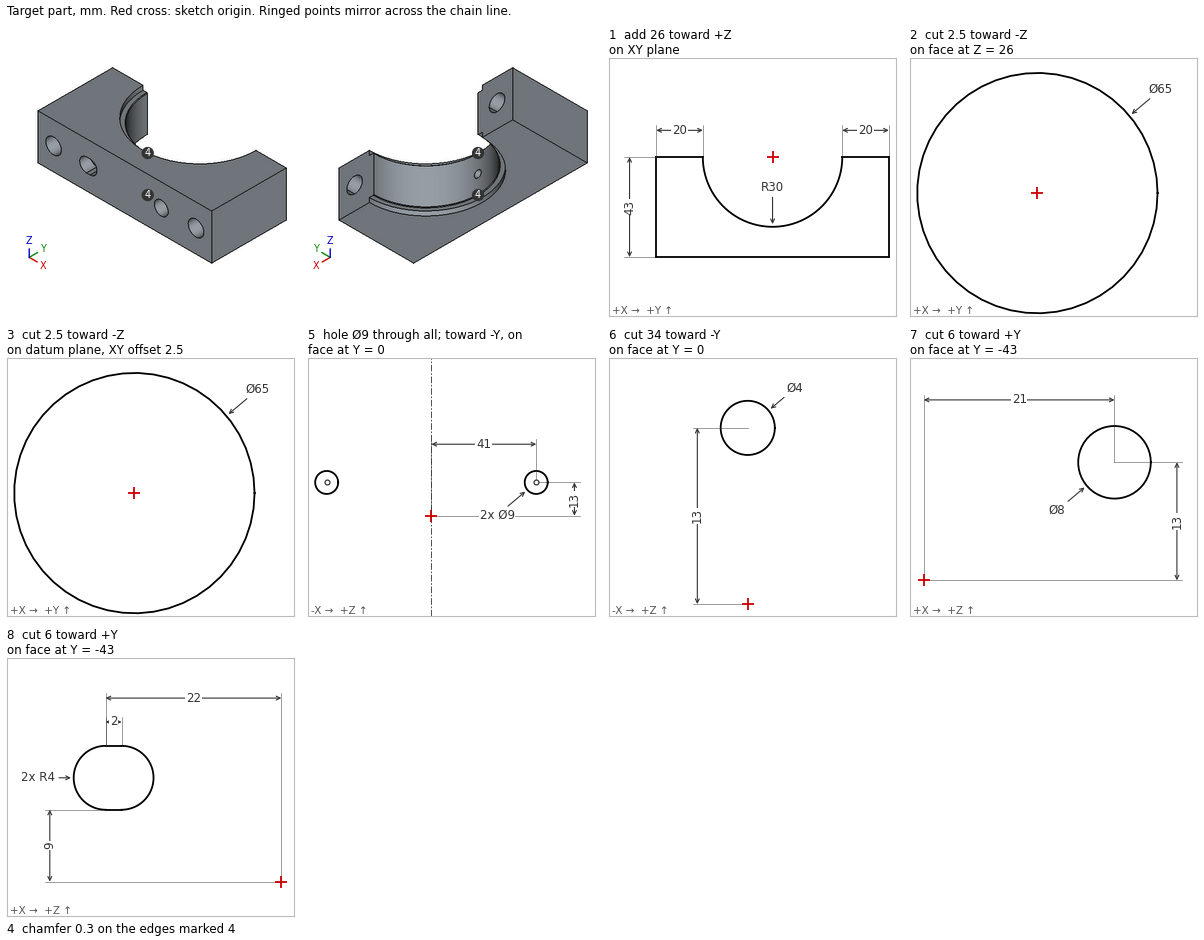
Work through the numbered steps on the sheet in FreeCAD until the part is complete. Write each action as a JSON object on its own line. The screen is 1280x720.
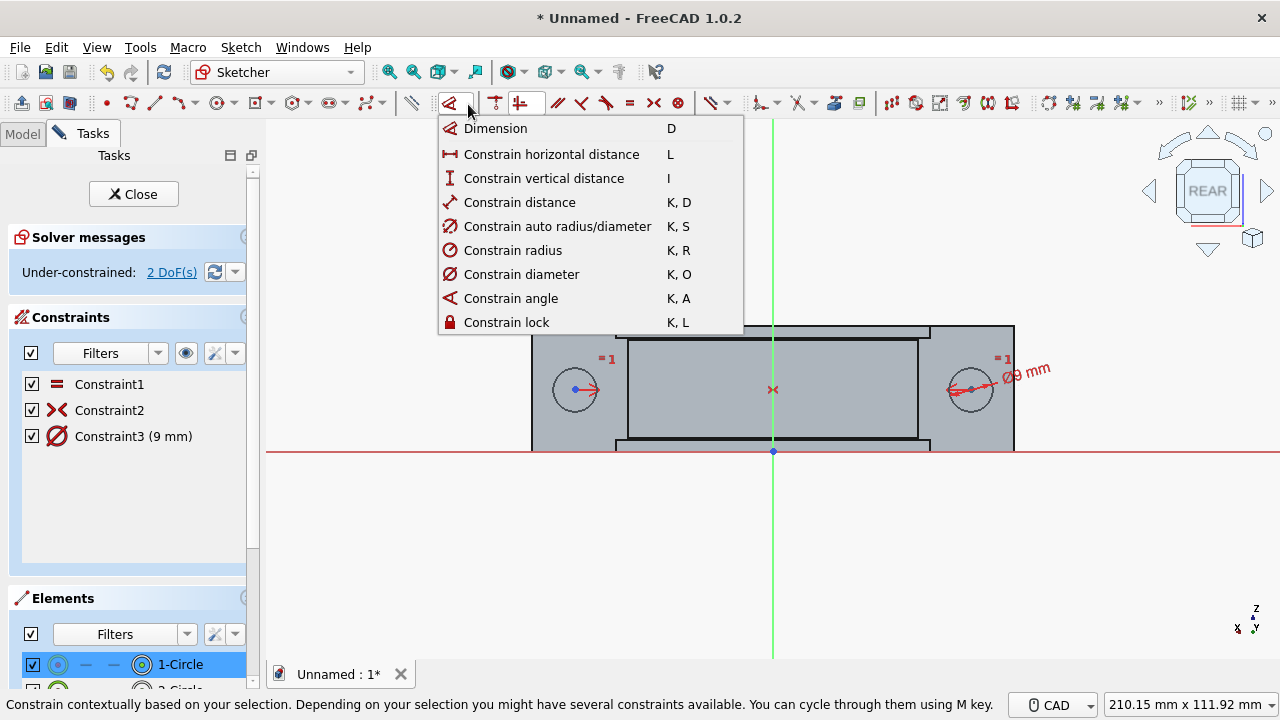
{"action": "left_click", "coordinate": [591, 154]}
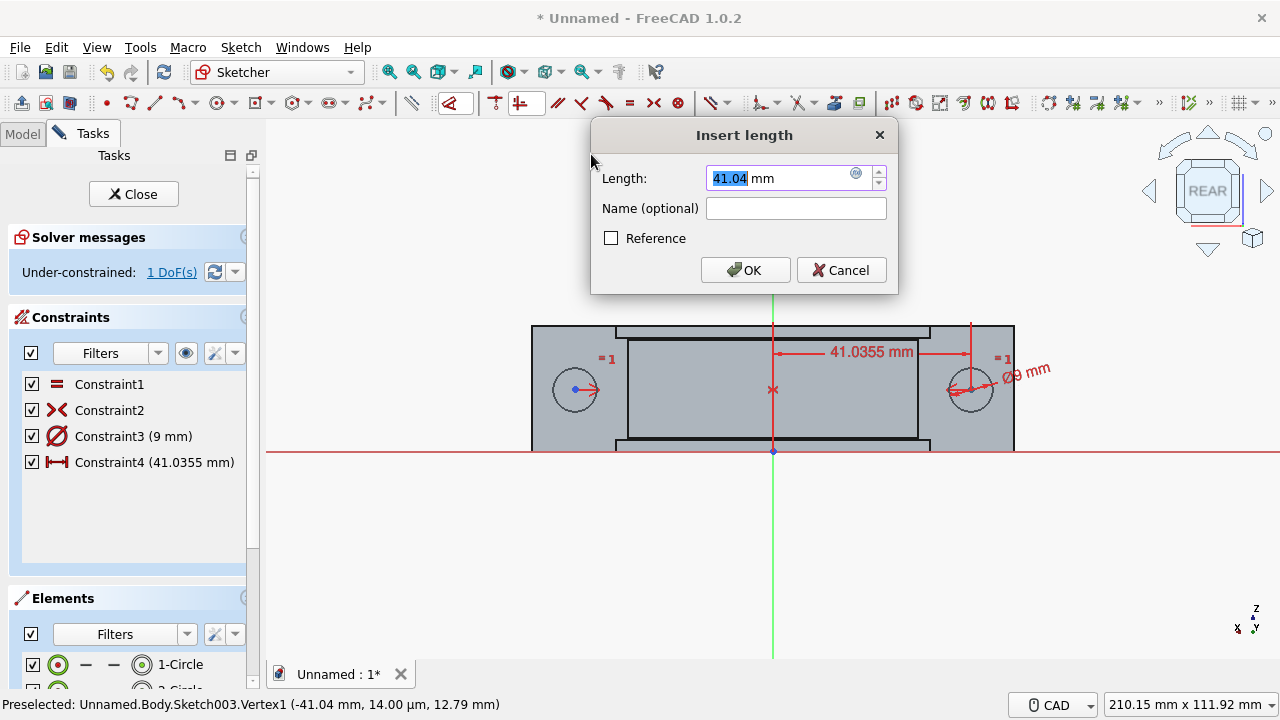
{"action": "type", "text": "41"}
{"action": "key", "text": "Return"}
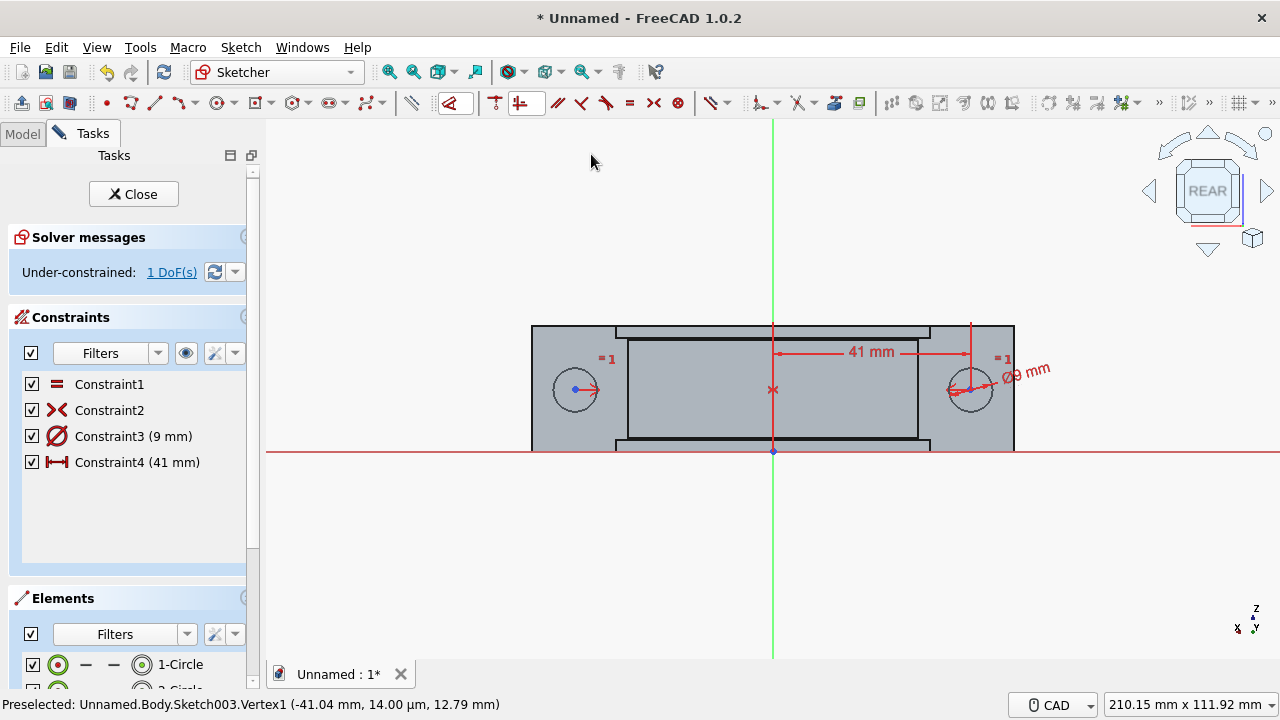
{"action": "left_click", "coordinate": [971, 390]}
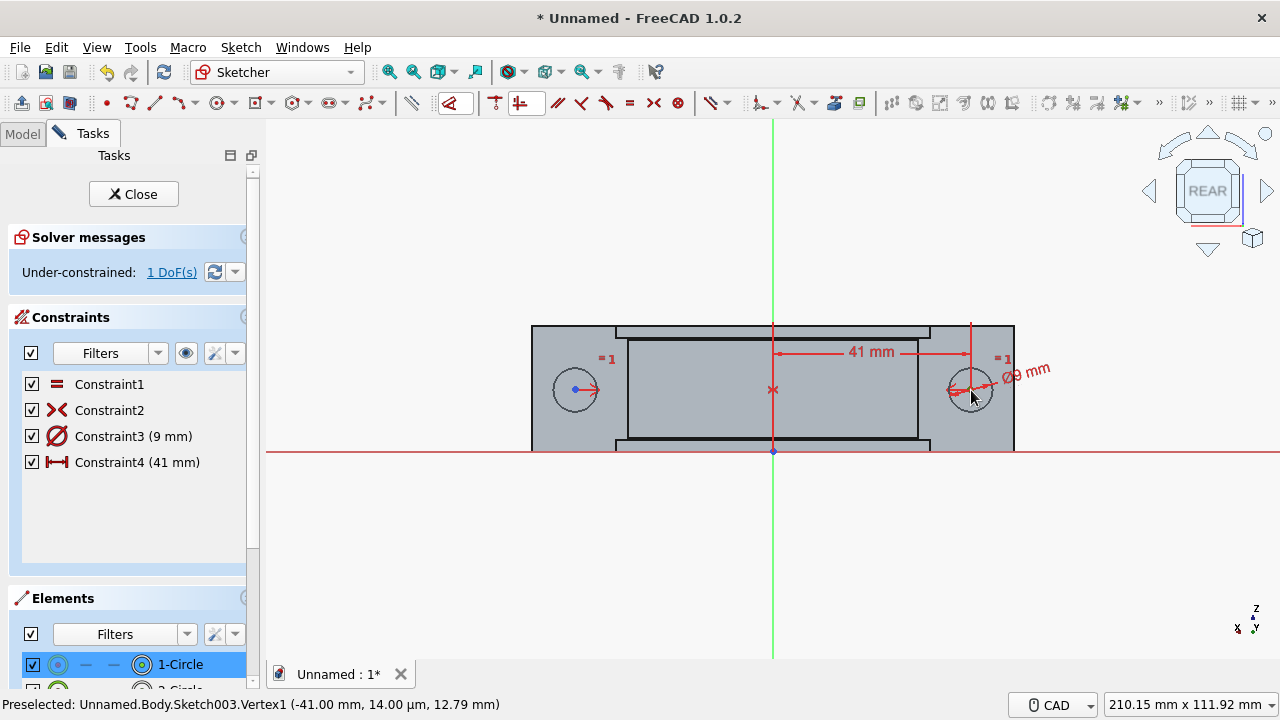
{"action": "left_click", "coordinate": [468, 104]}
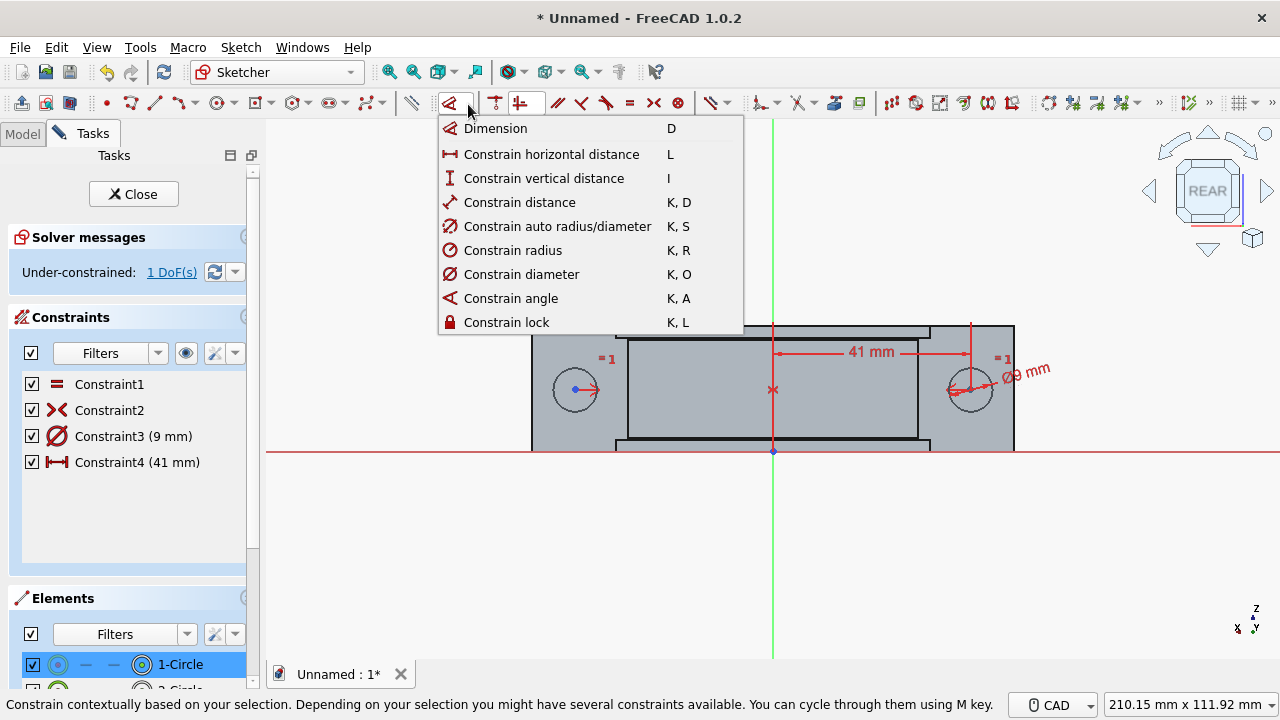
{"action": "left_click", "coordinate": [591, 178]}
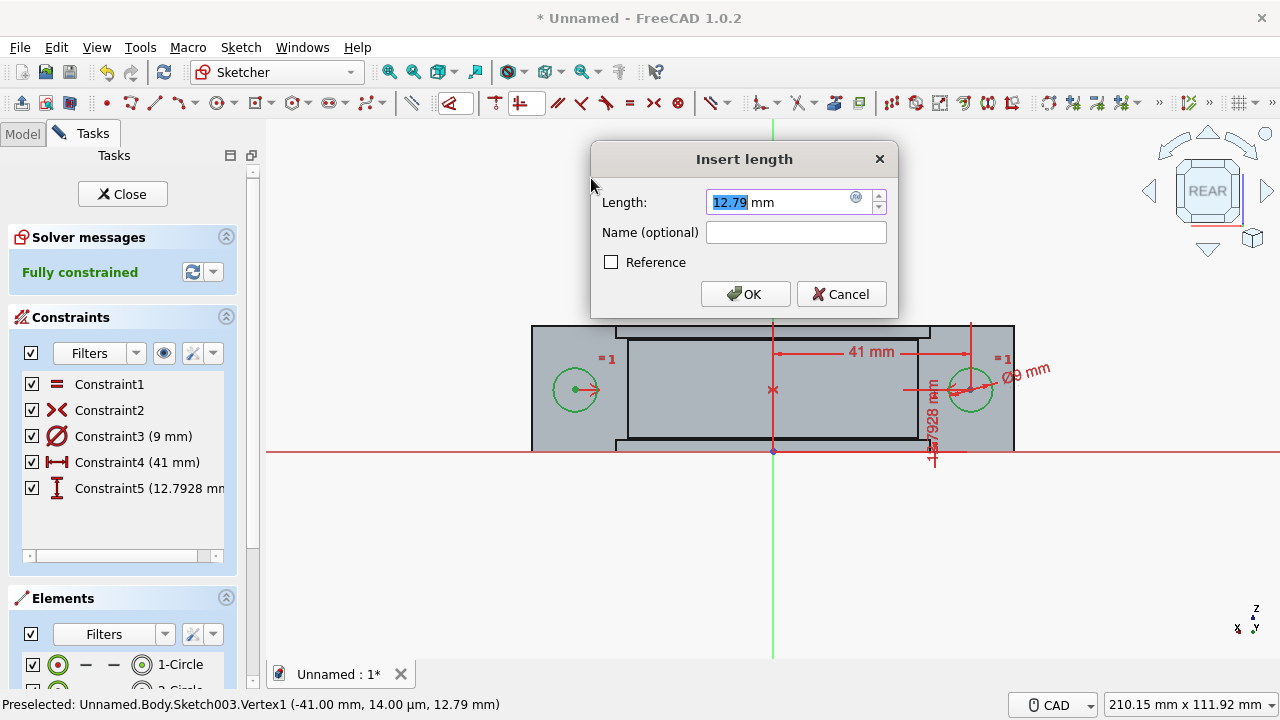
{"action": "type", "text": "13"}
{"action": "key", "text": "Return"}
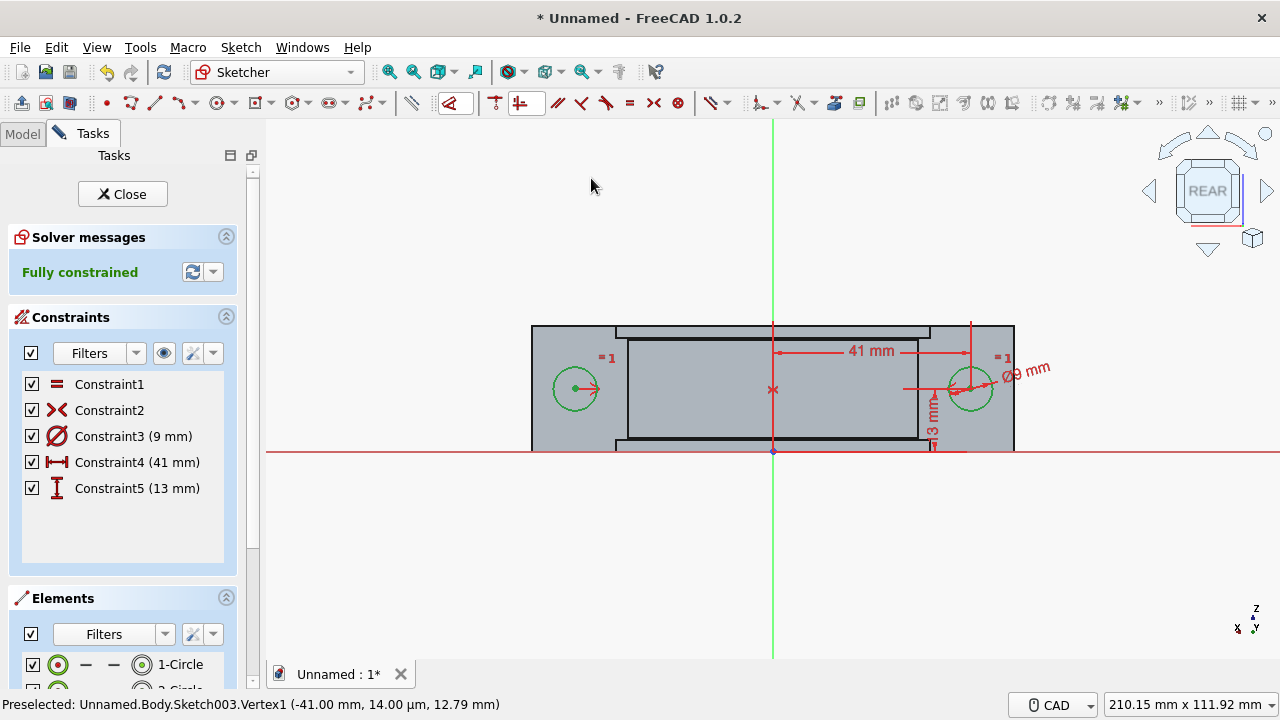
{"action": "left_click", "coordinate": [123, 194]}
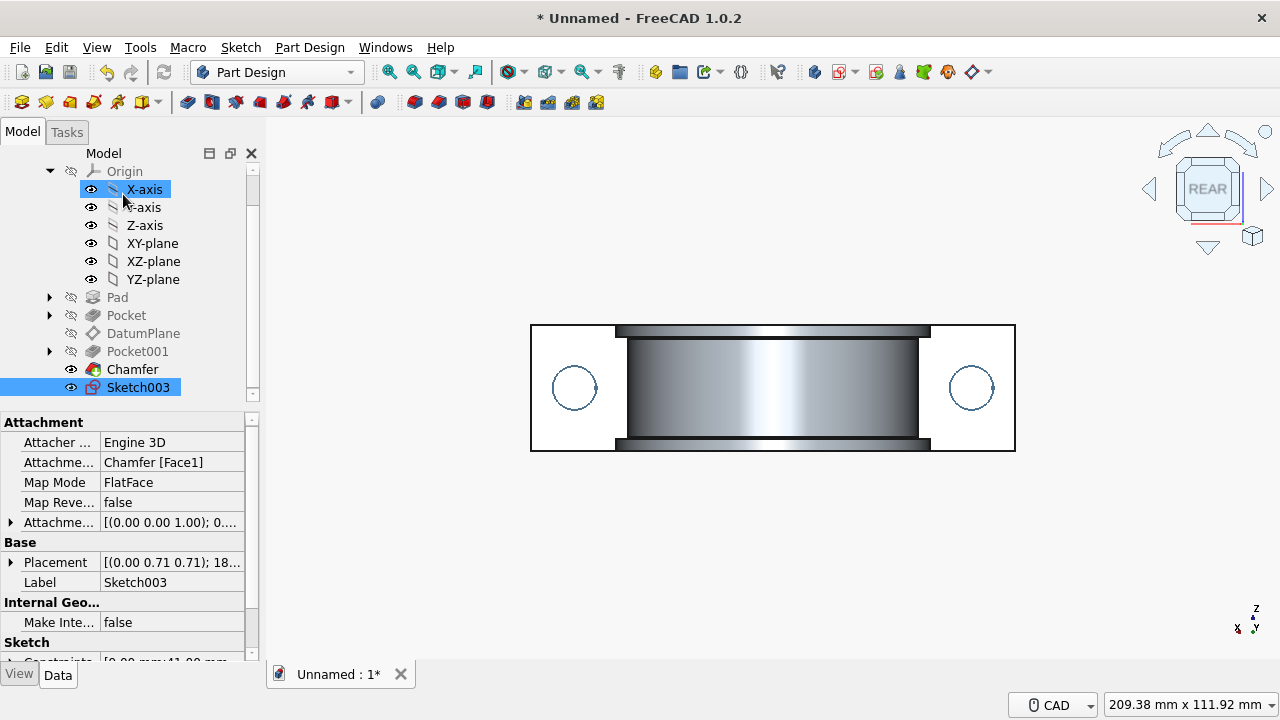
{"action": "left_click", "coordinate": [212, 102]}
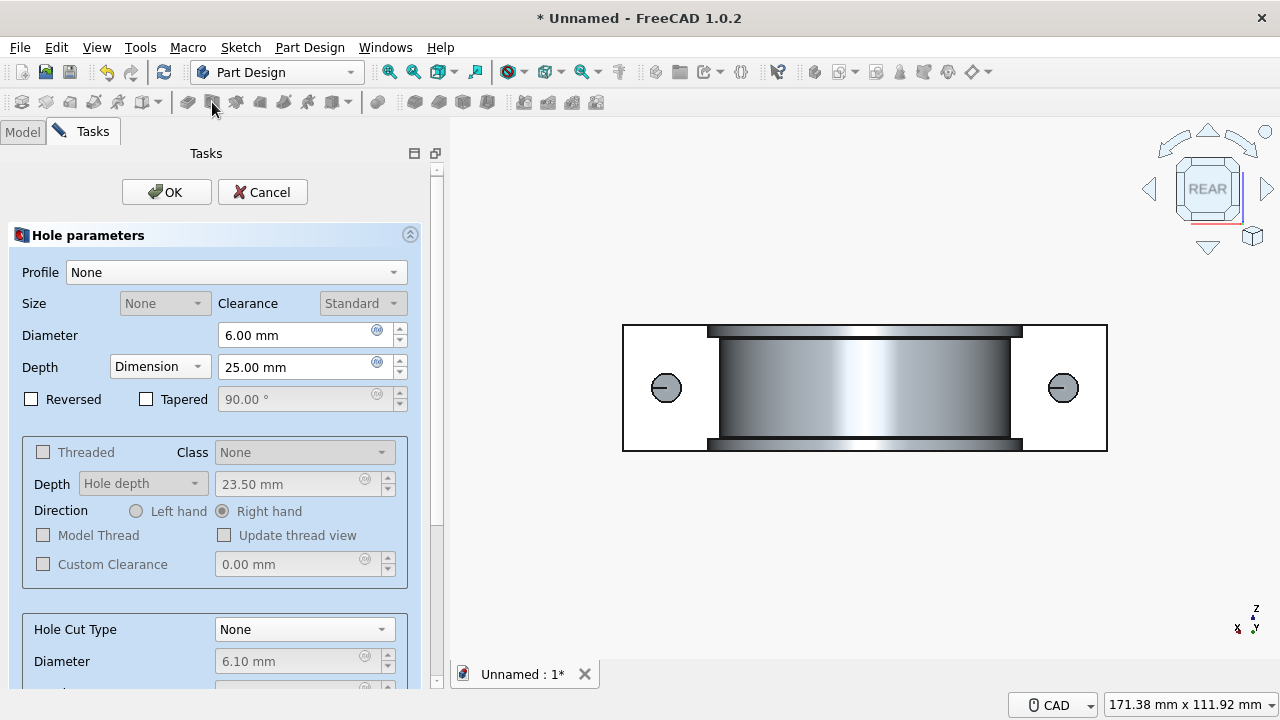
{"action": "triple_click", "coordinate": [305, 335]}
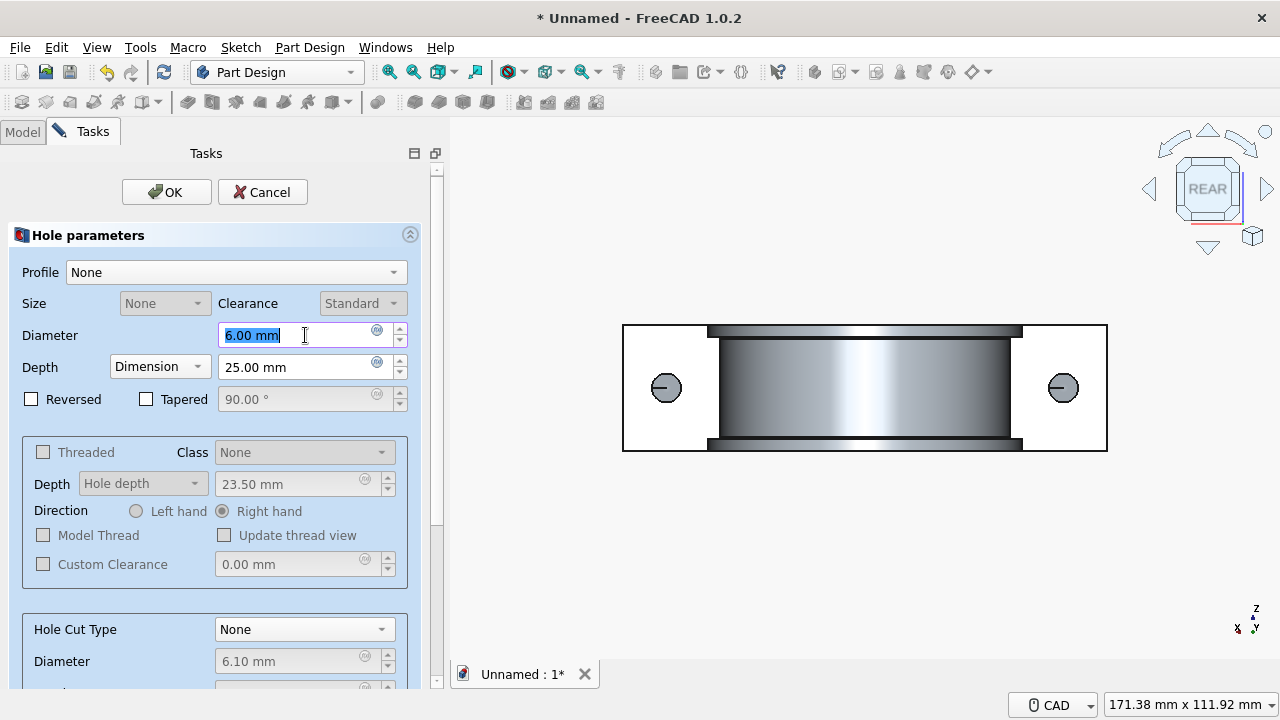
{"action": "type", "text": "9"}
{"action": "key", "text": "Tab"}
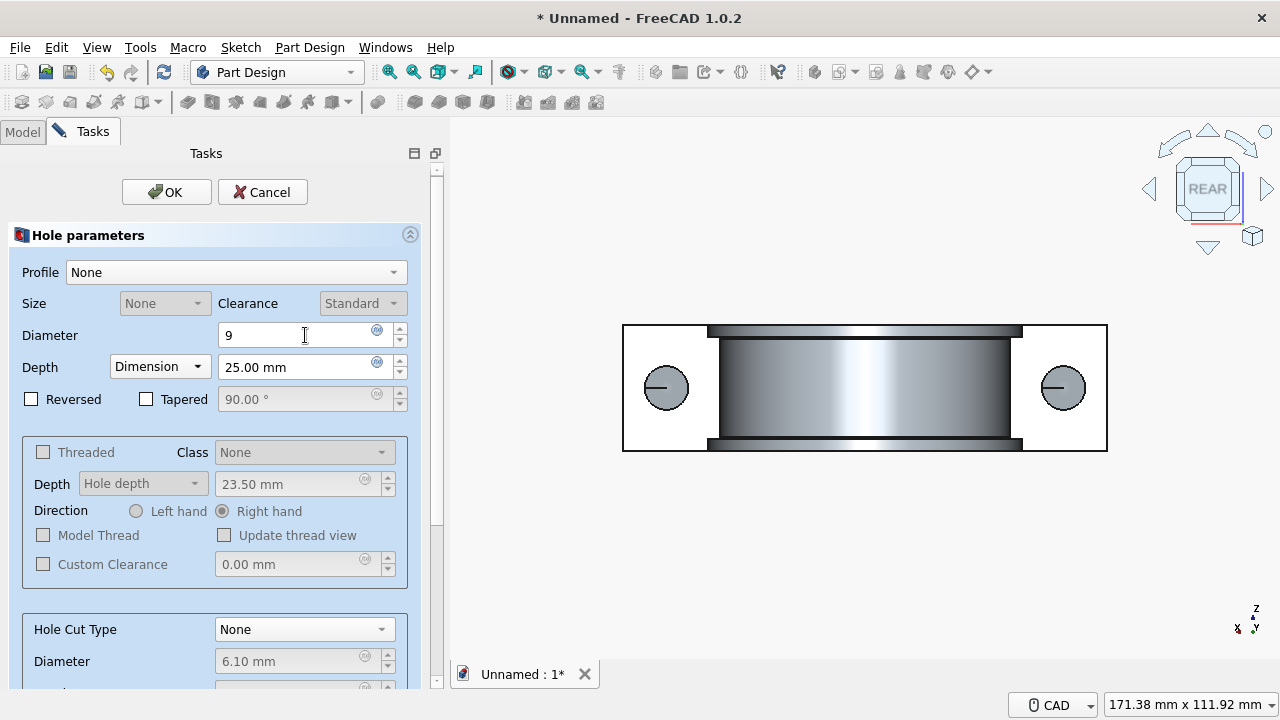
{"action": "left_click", "coordinate": [161, 366]}